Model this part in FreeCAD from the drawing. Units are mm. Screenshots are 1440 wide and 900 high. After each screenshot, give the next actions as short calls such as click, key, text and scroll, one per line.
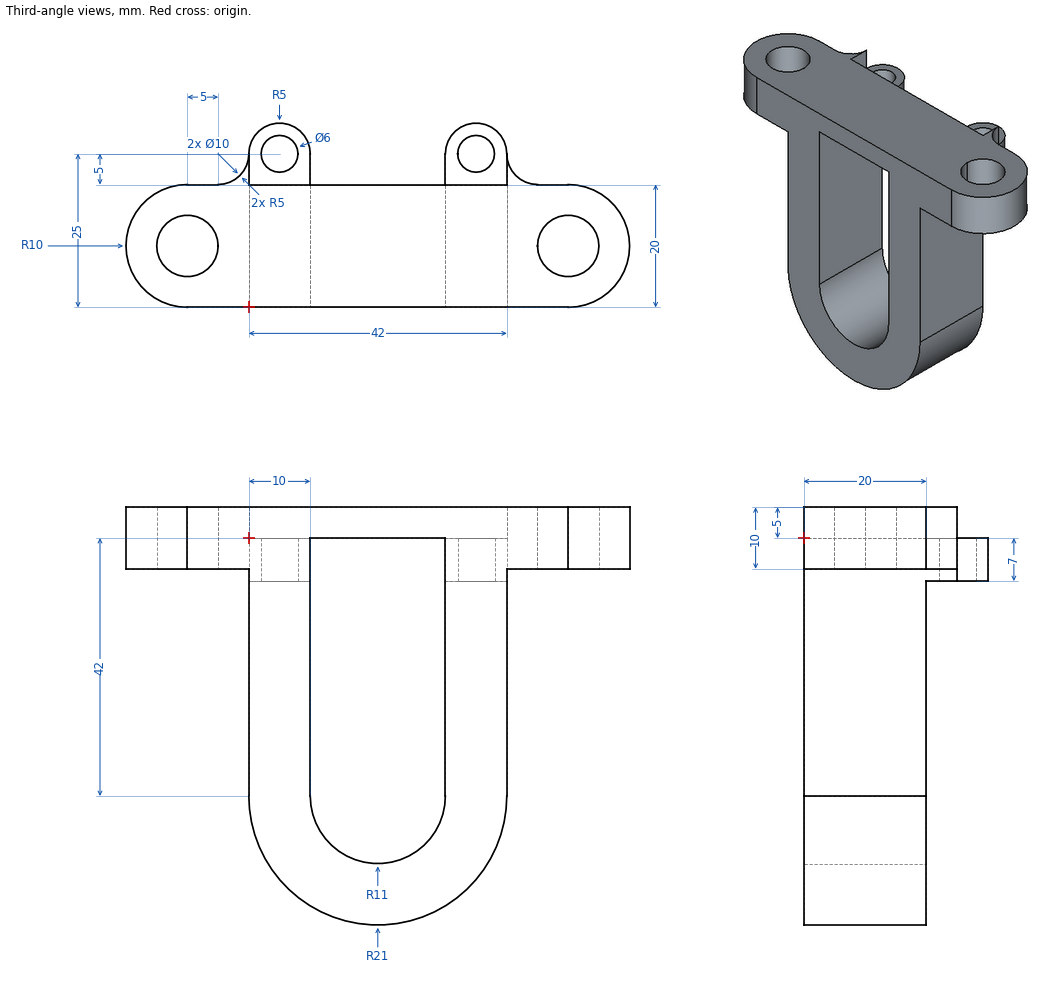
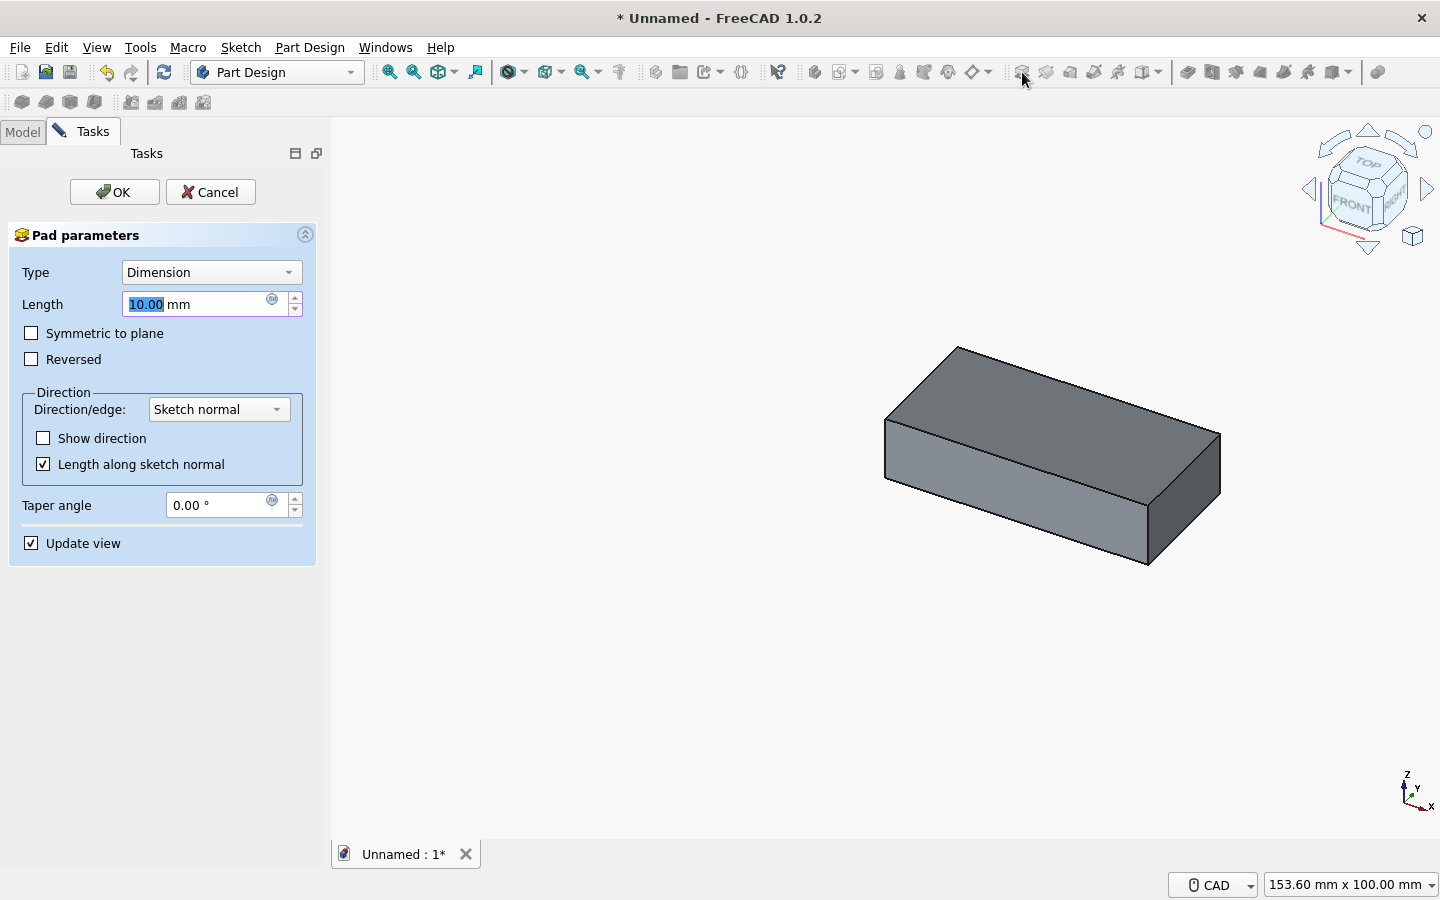
text(5)
key(Tab)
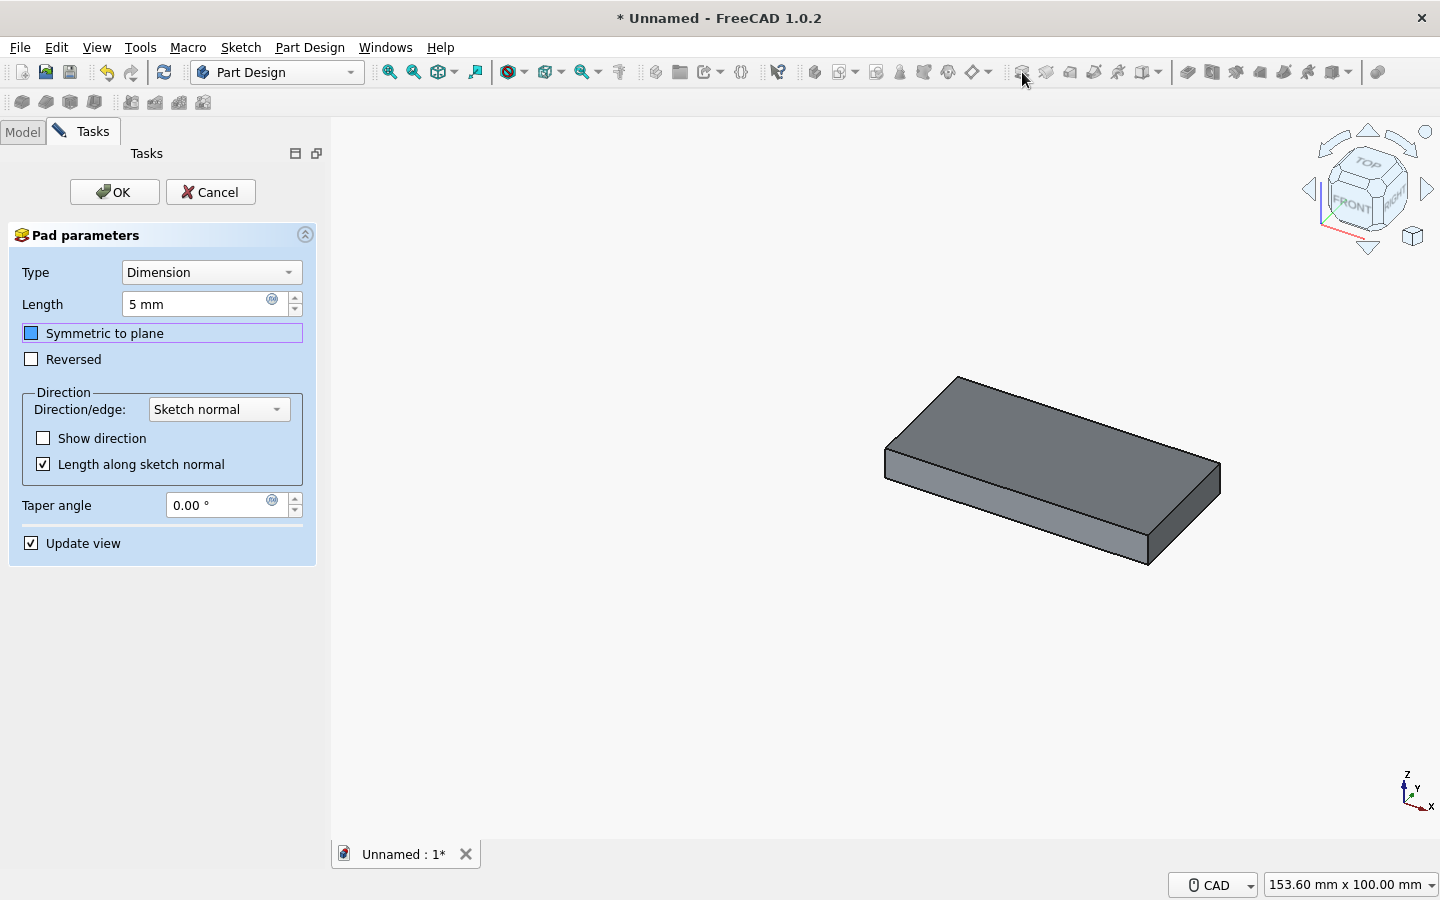
click(115, 192)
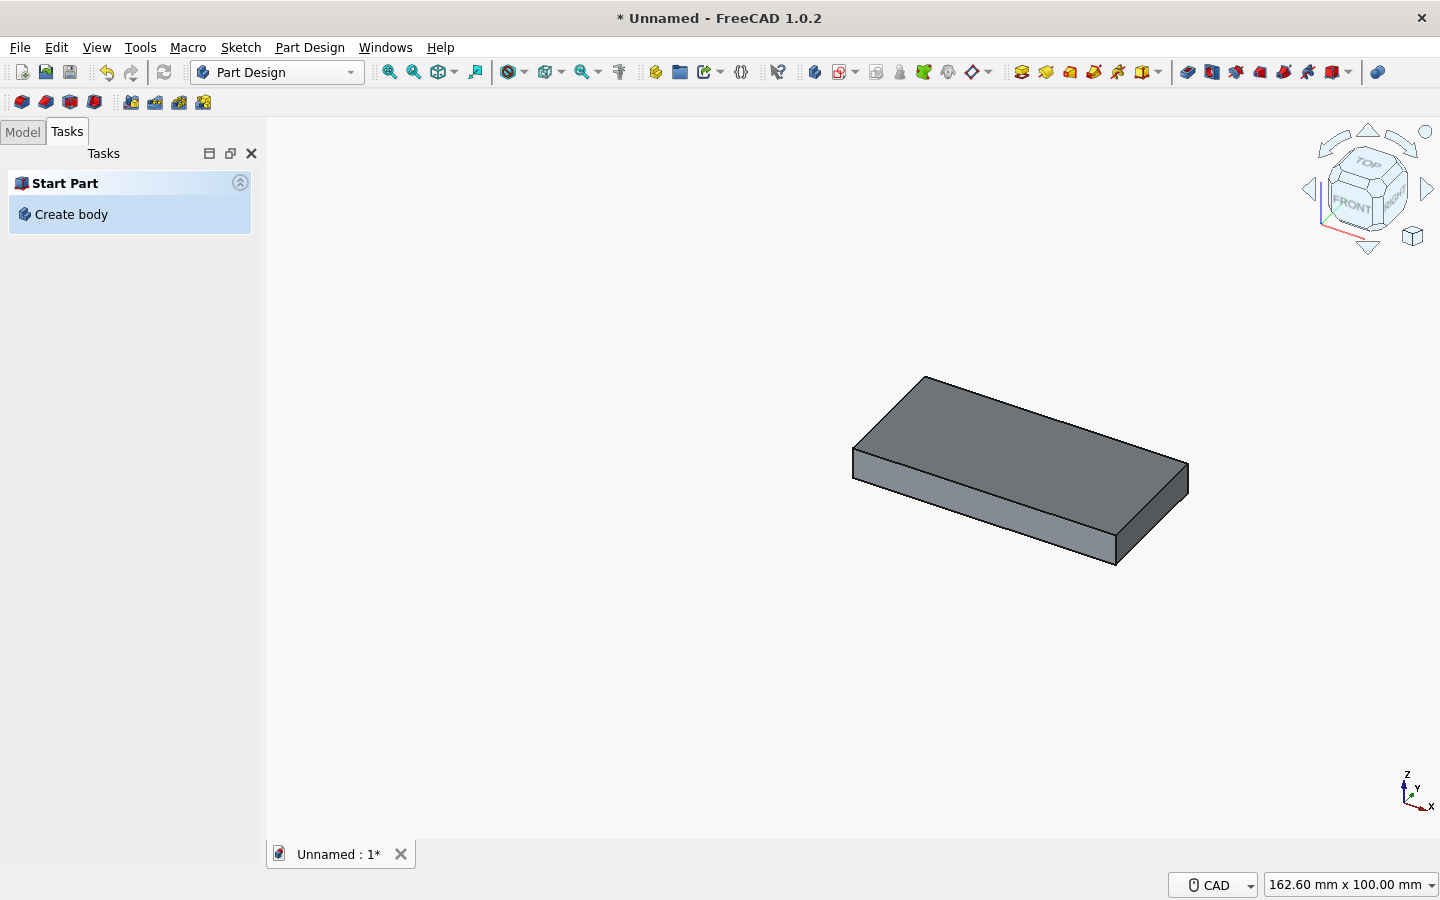
click(390, 72)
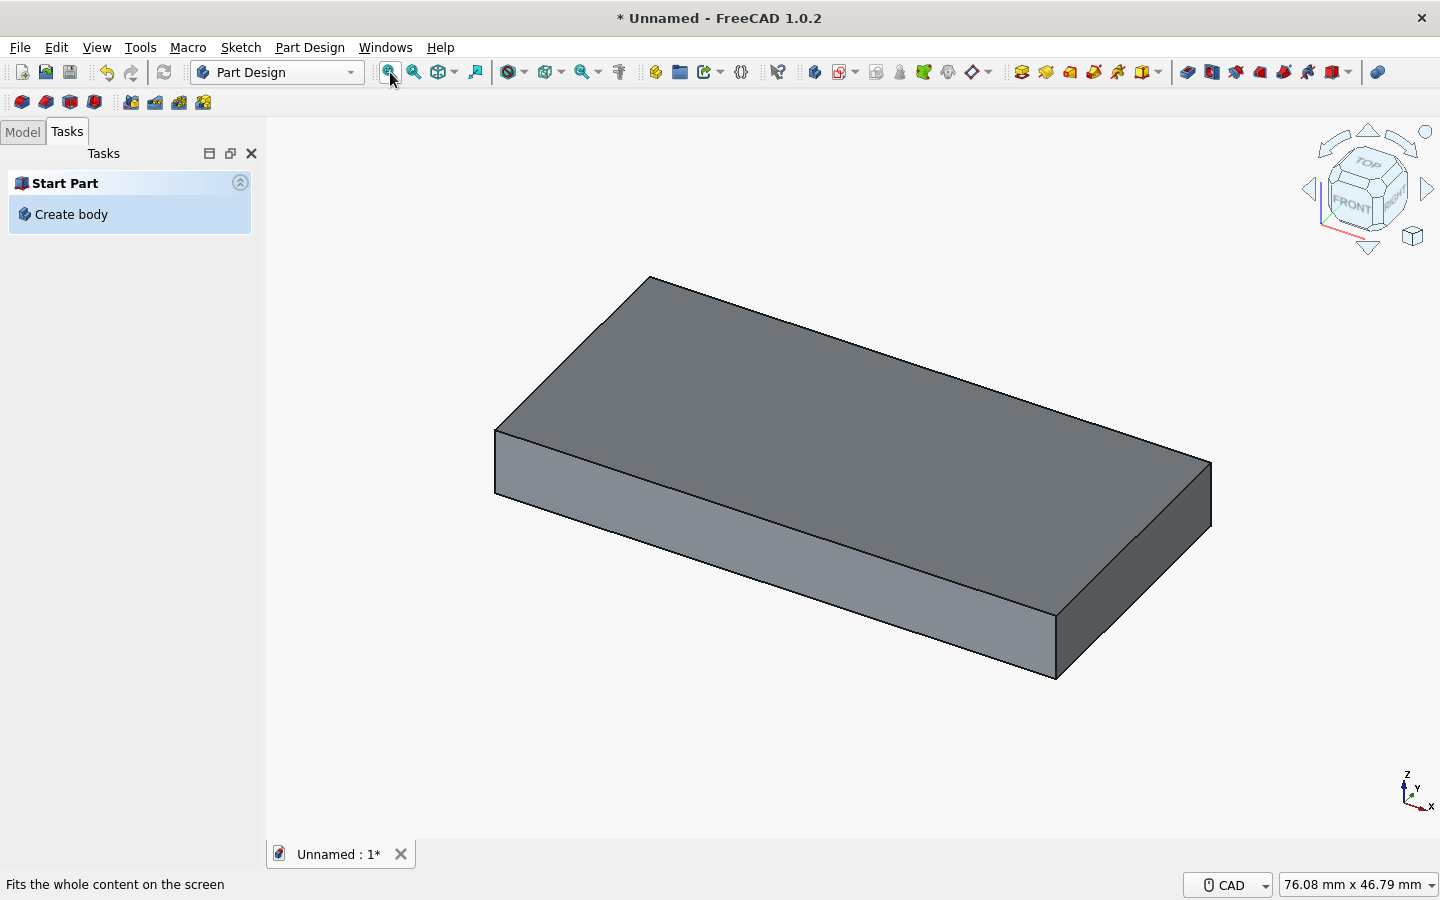
key(4)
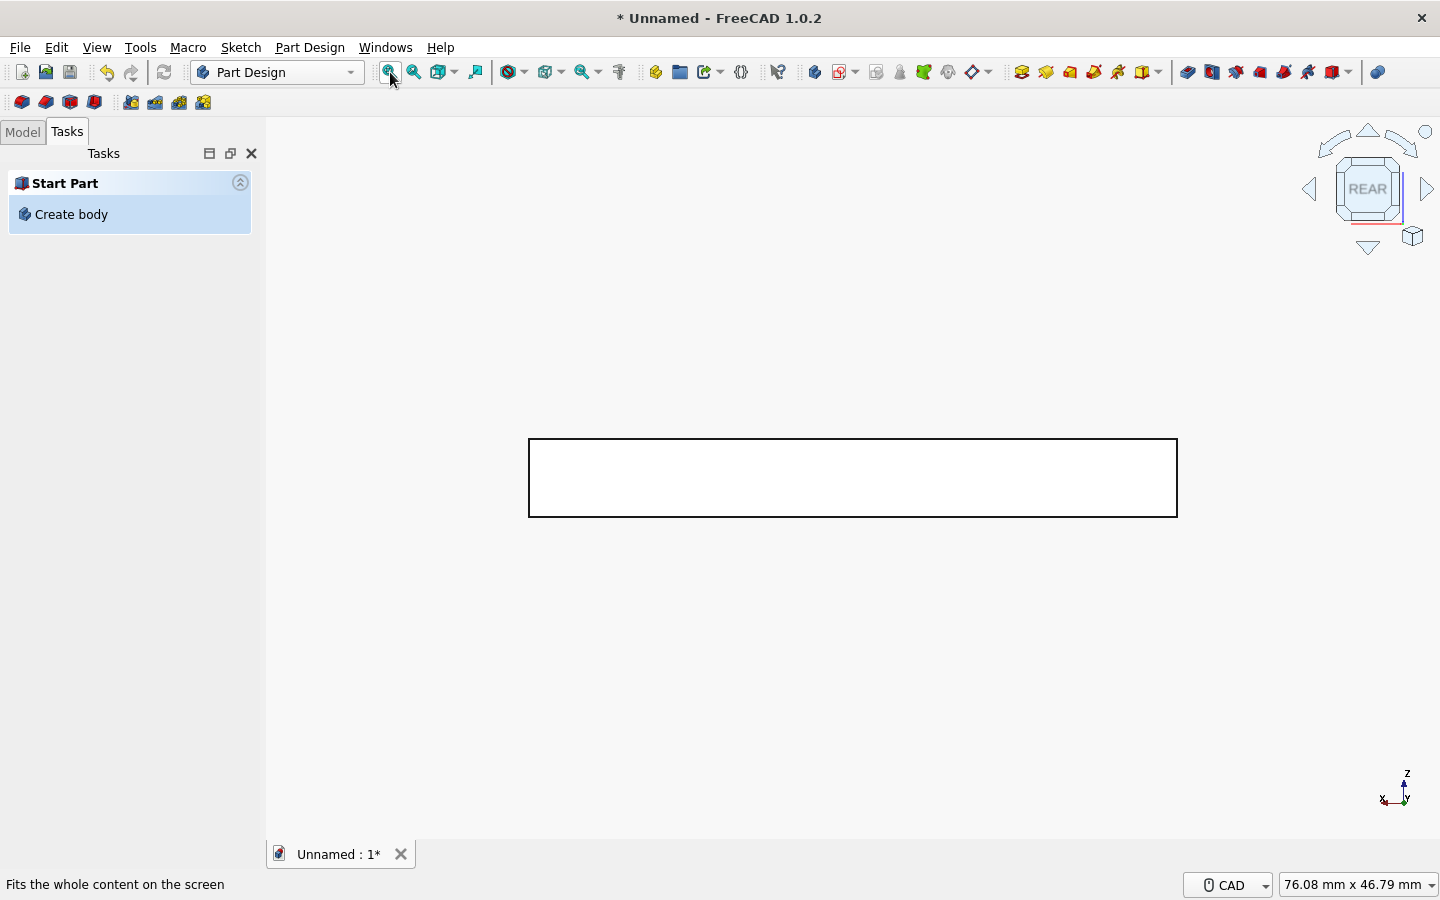
click(575, 477)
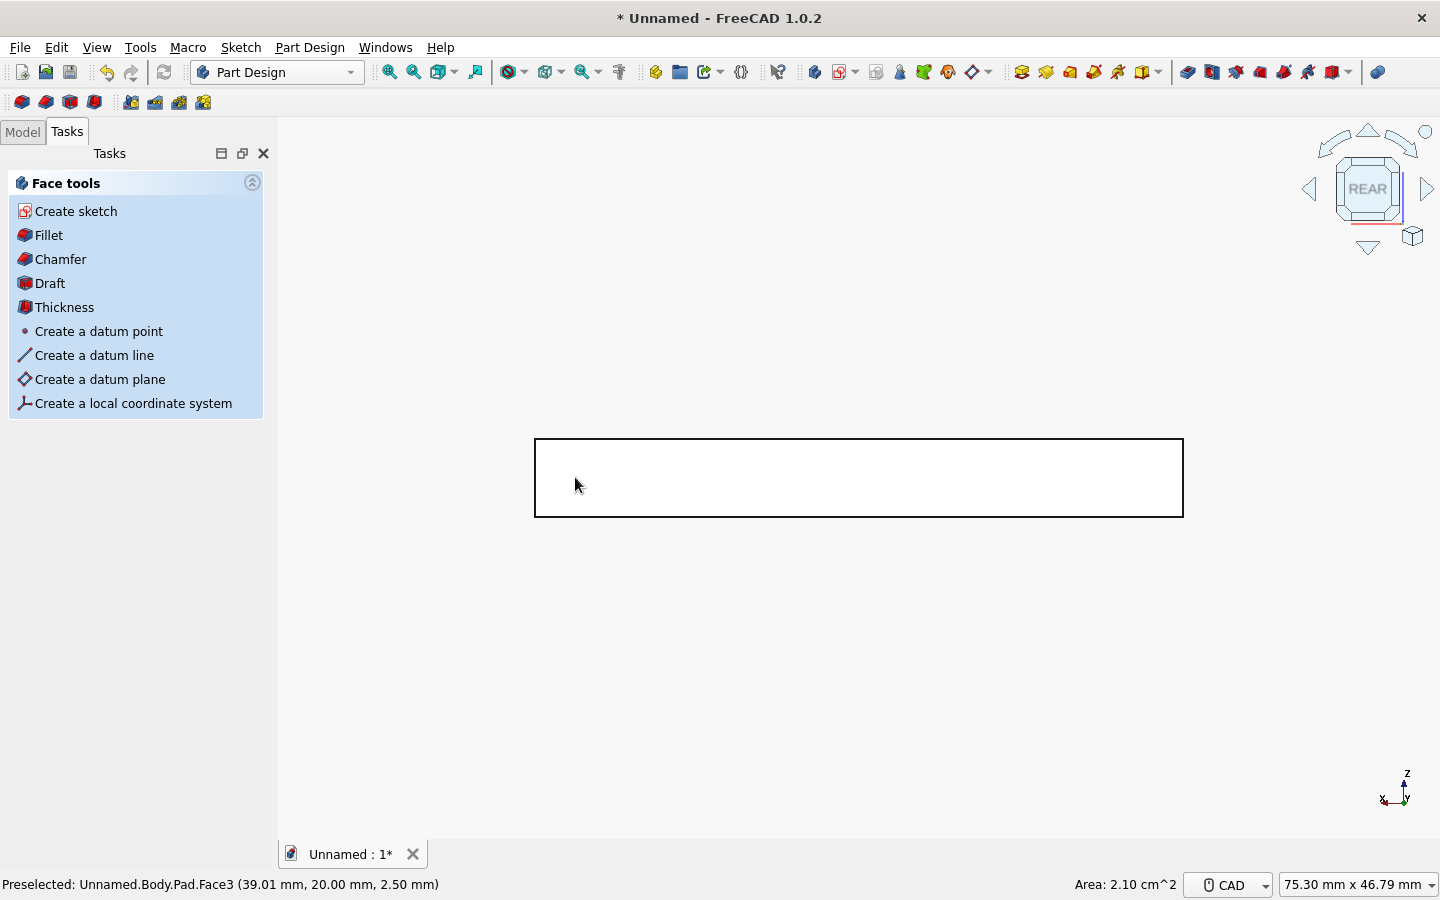
click(840, 72)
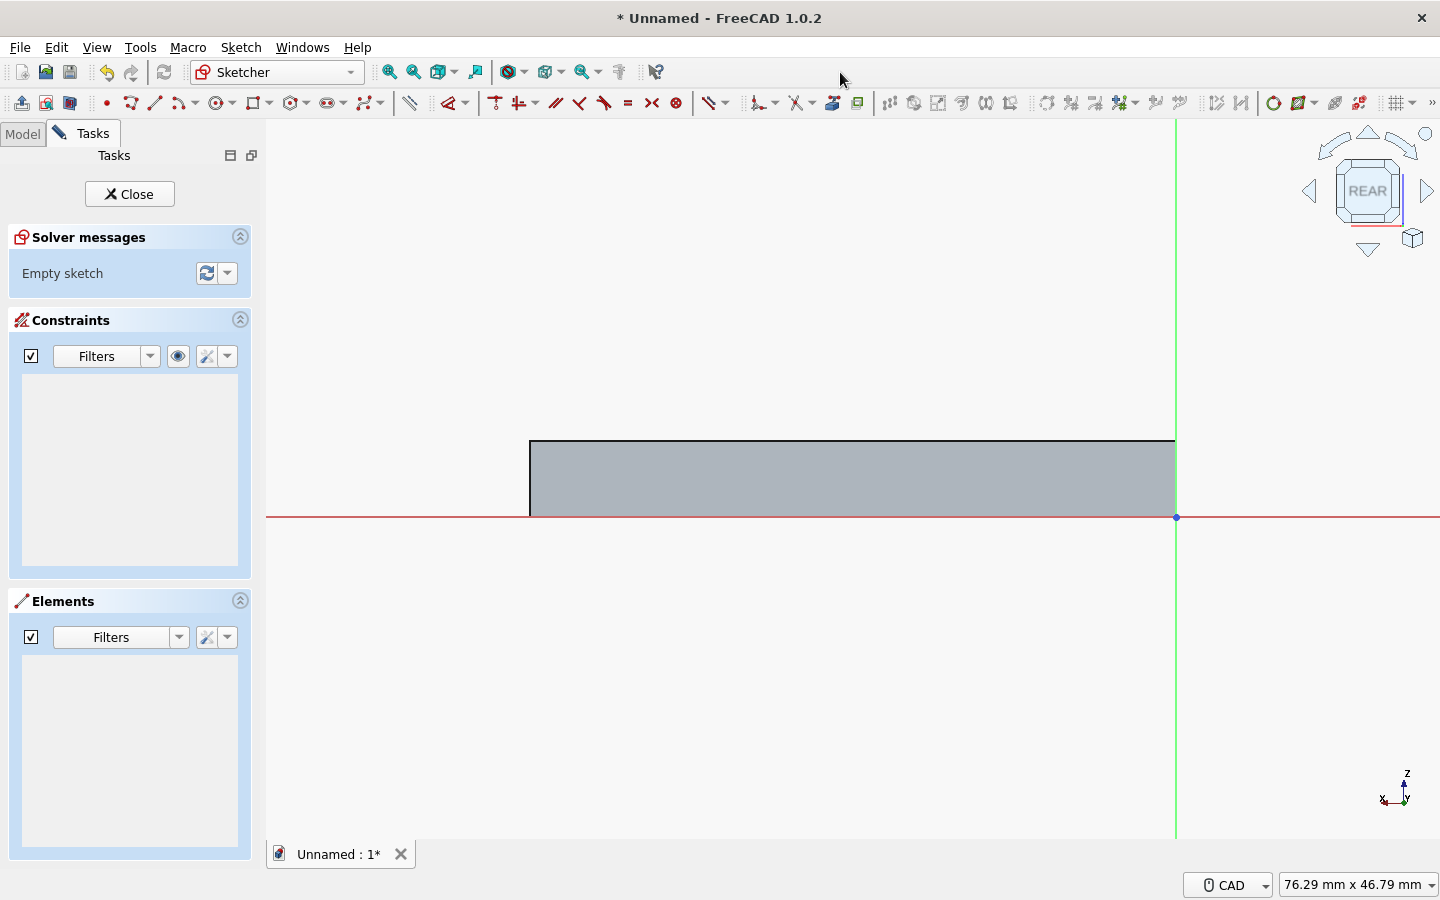
scroll(729, 147, down, 4)